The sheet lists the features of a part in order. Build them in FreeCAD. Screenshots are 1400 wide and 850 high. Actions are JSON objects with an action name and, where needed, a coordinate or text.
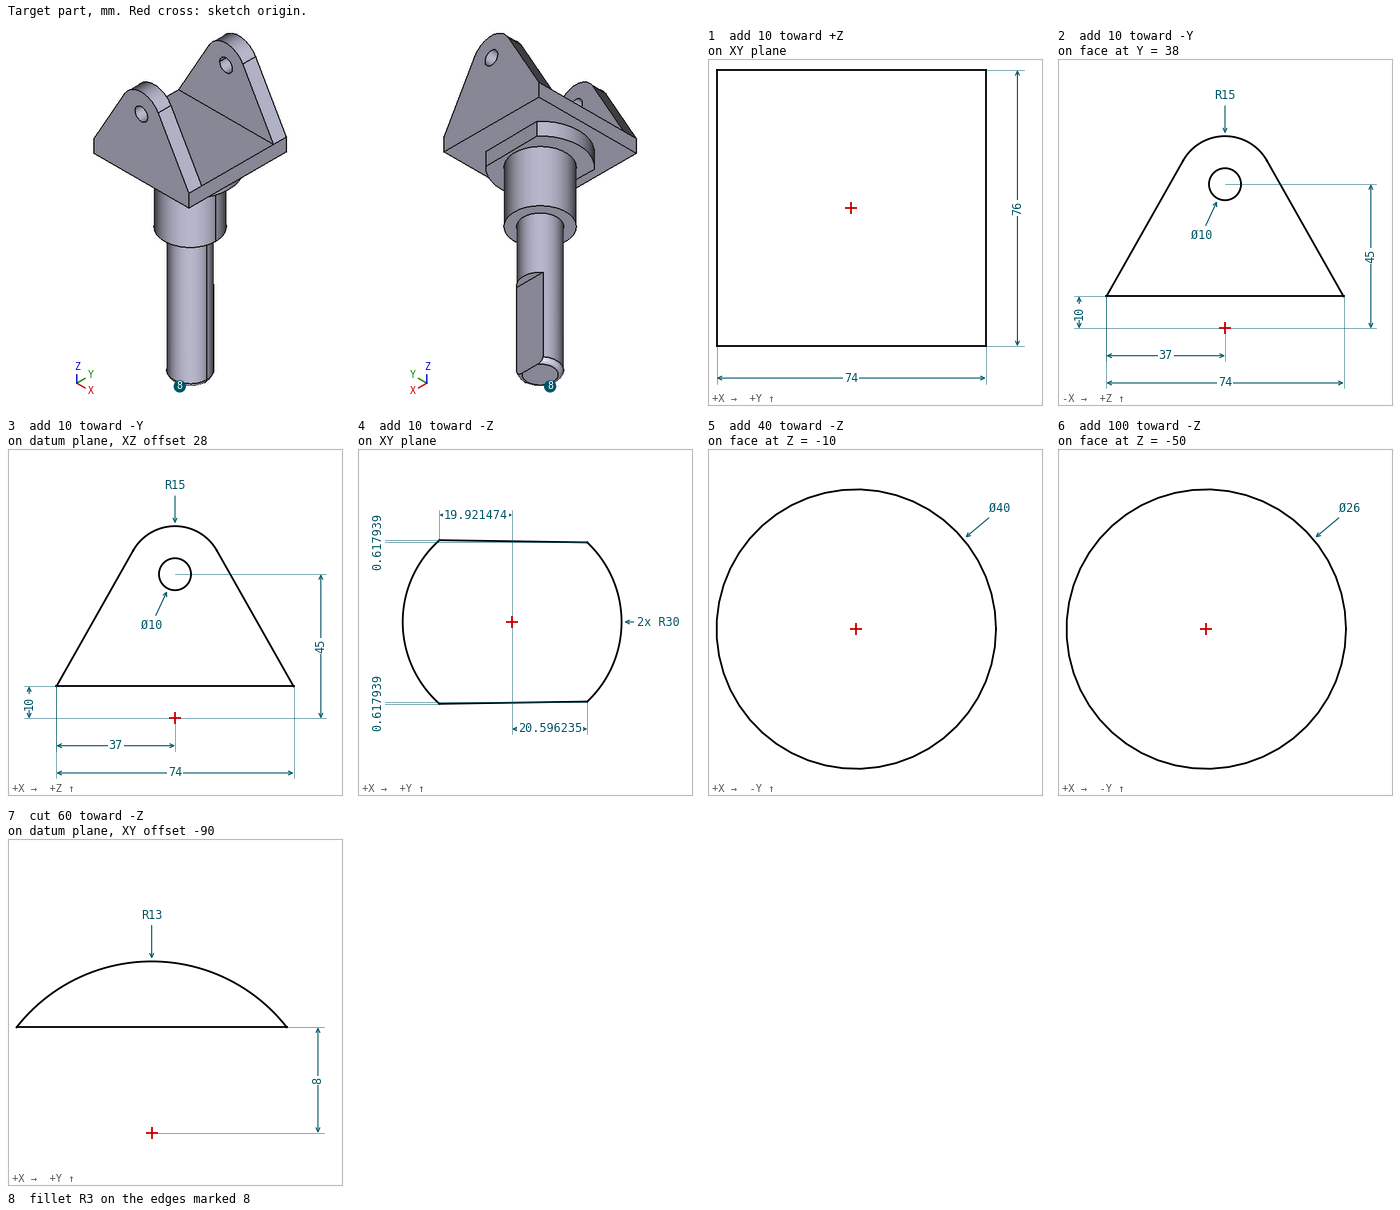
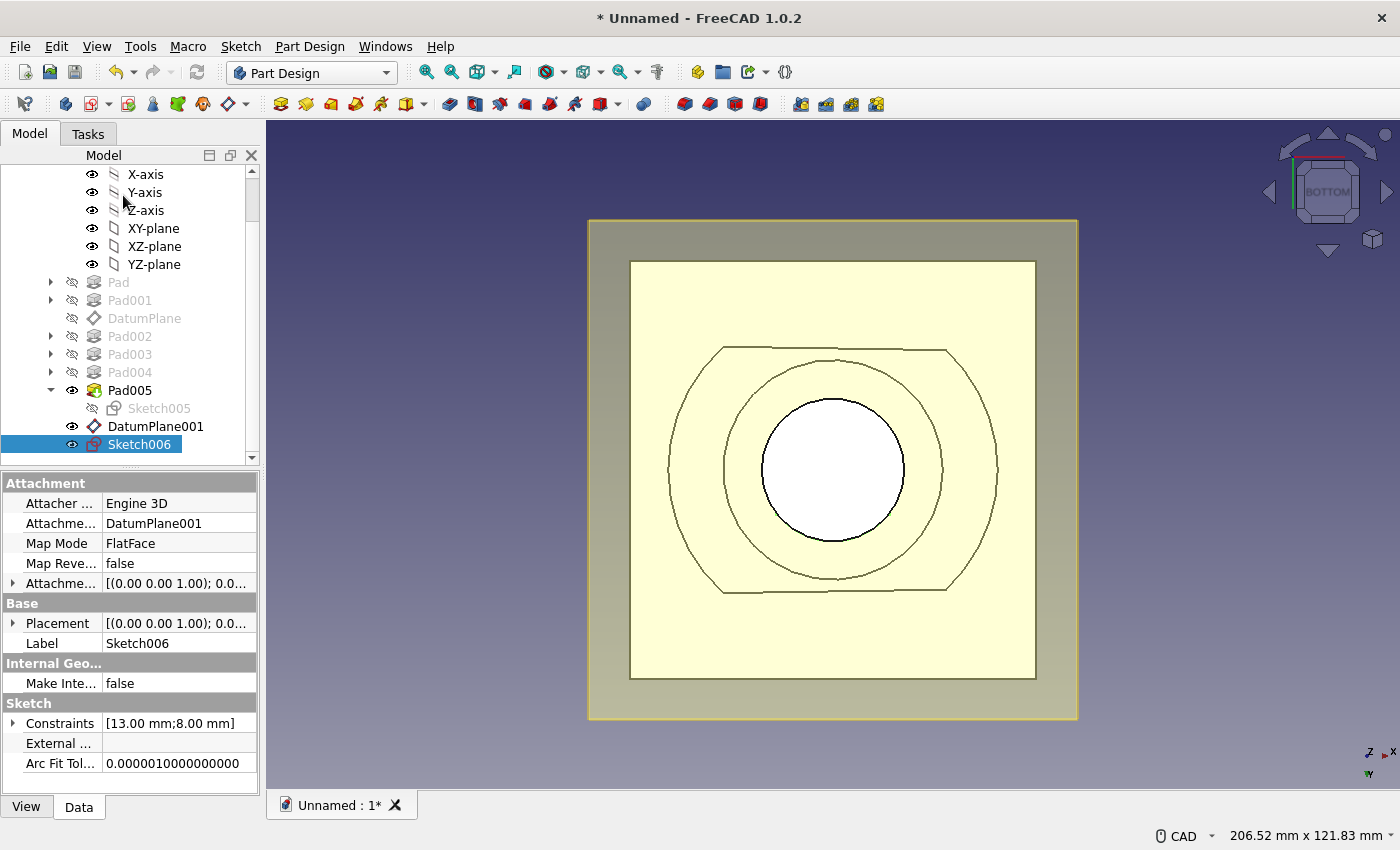
{"action": "left_click", "coordinate": [450, 104]}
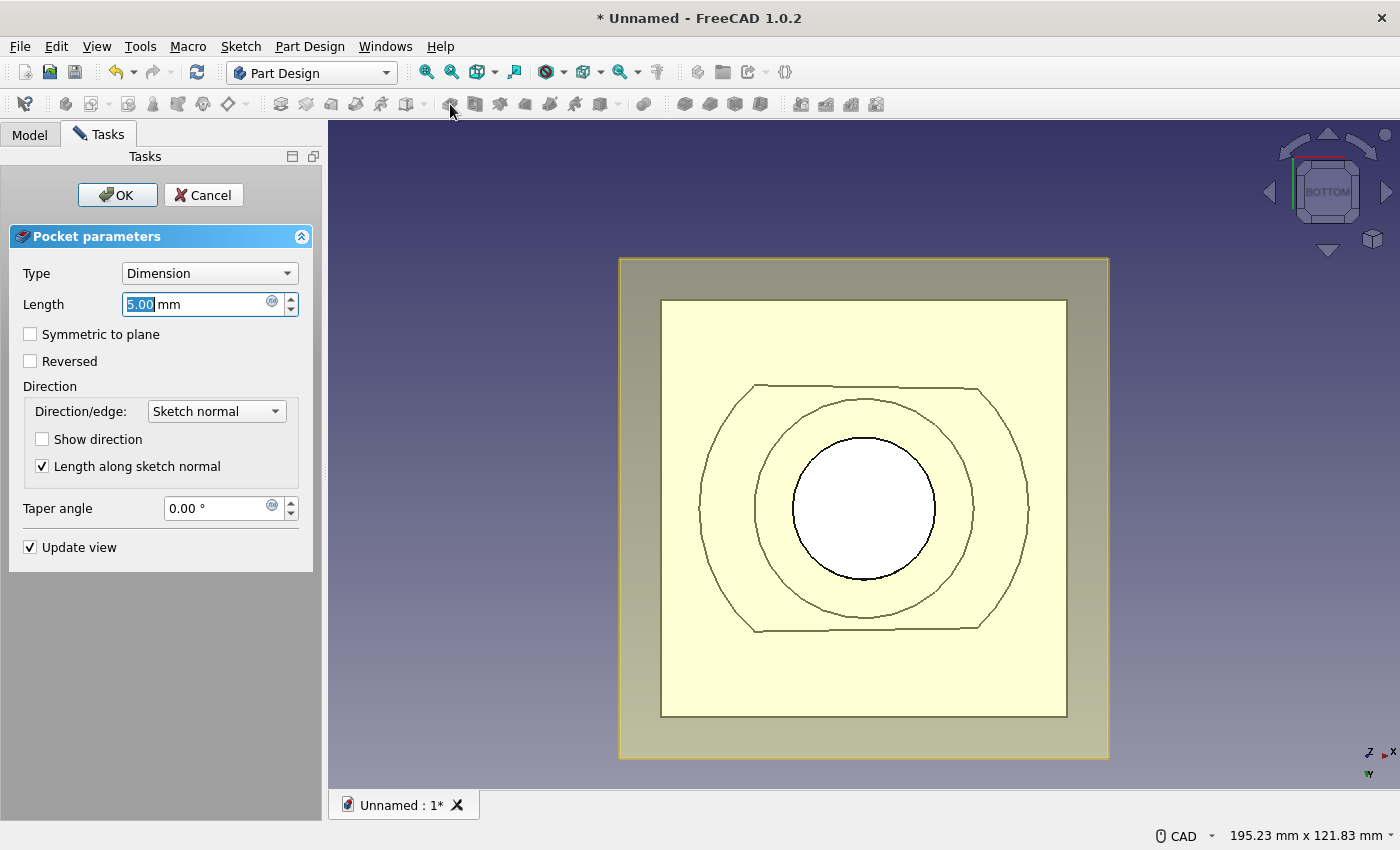
{"action": "type", "text": "60"}
{"action": "key", "text": "Tab"}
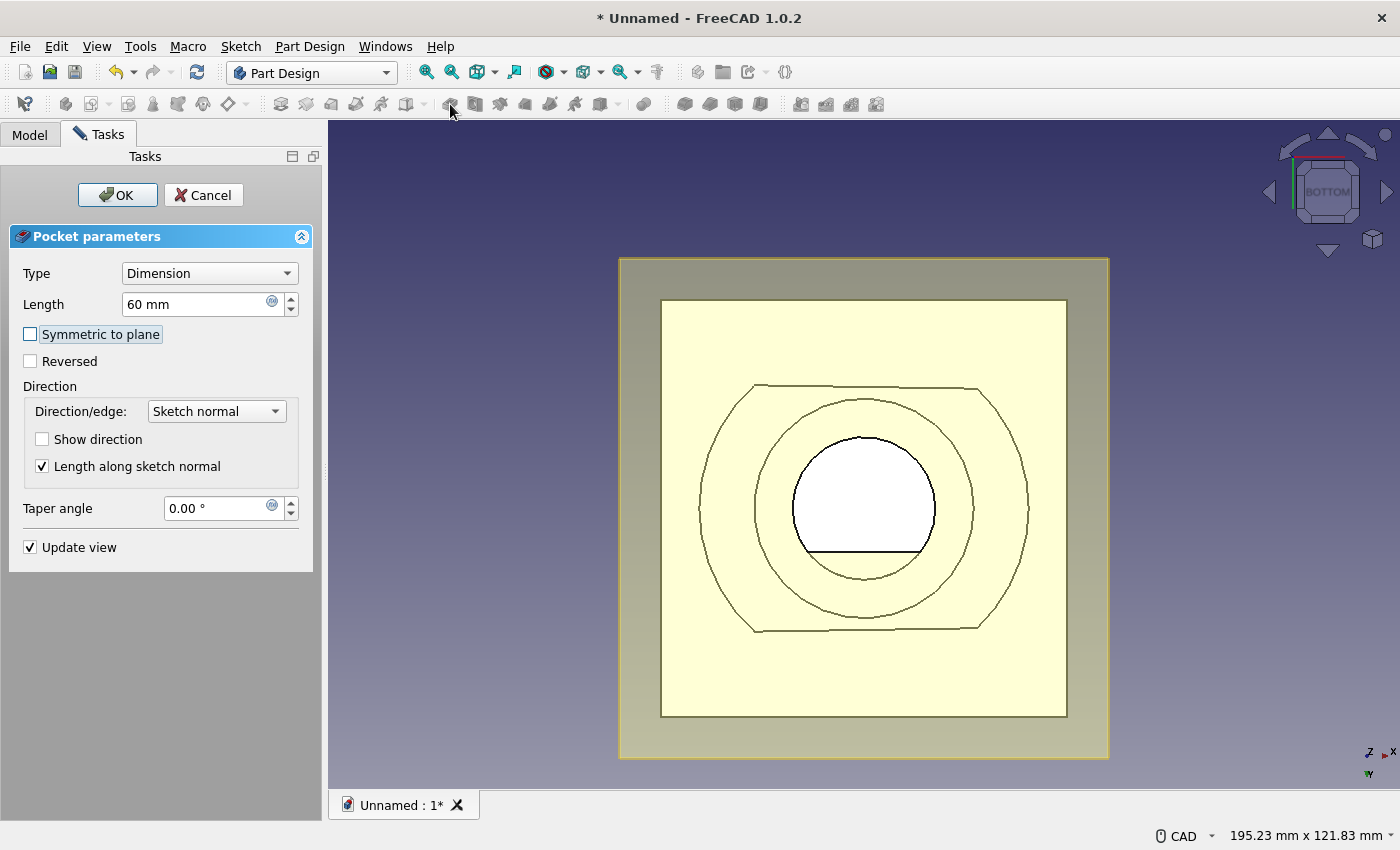
{"action": "left_click", "coordinate": [118, 195]}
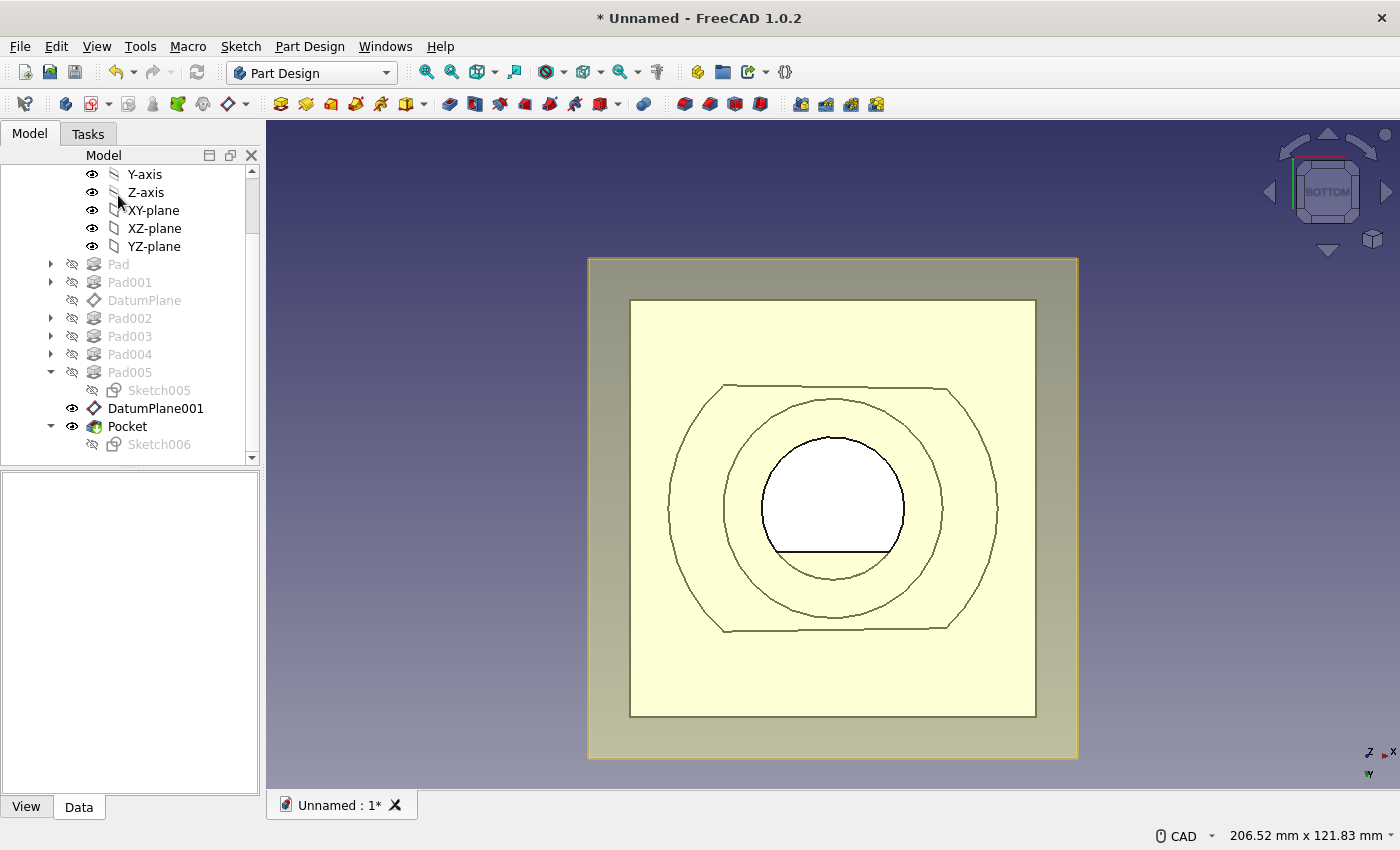
{"action": "left_click", "coordinate": [117, 408]}
{"action": "key", "text": "space"}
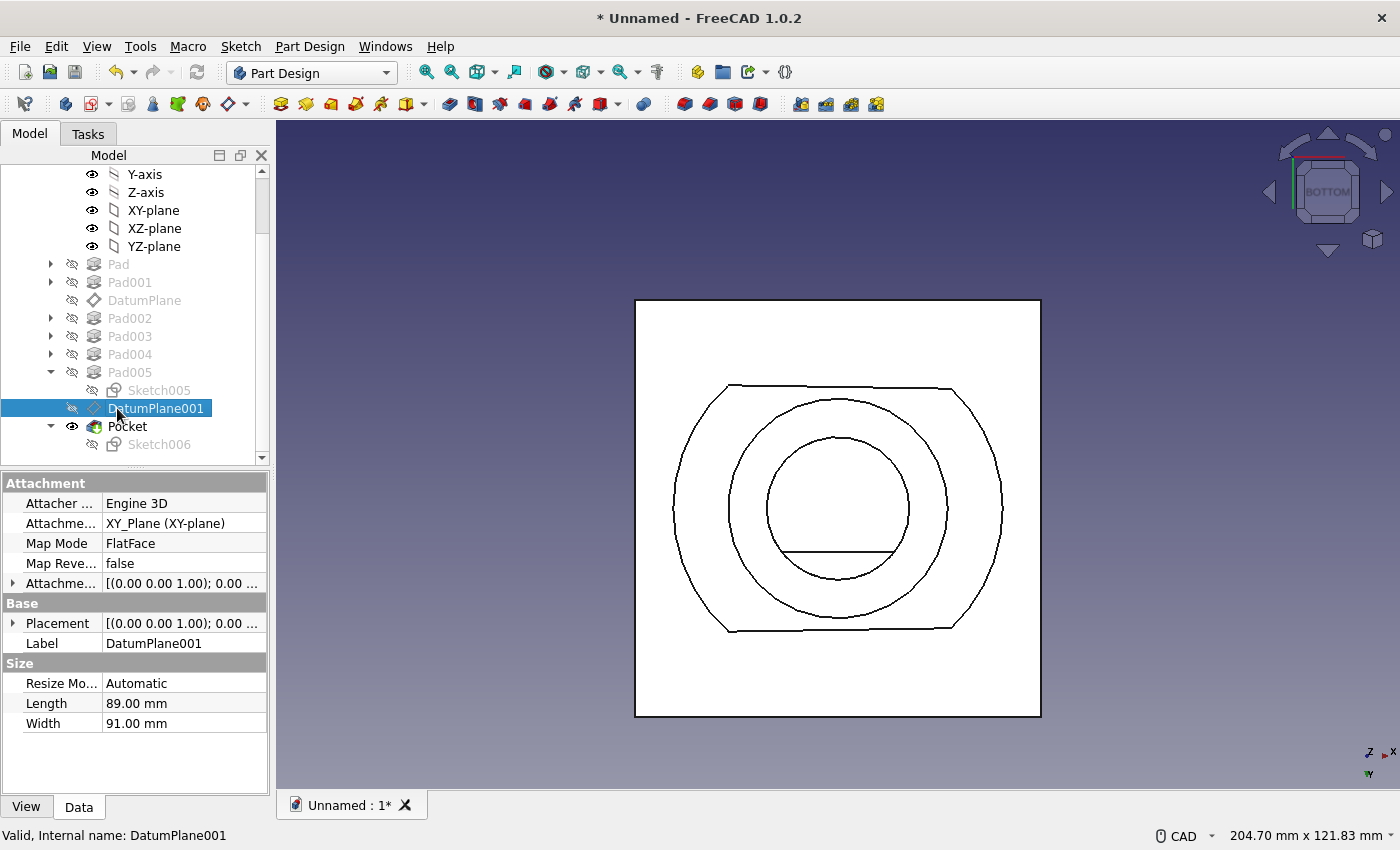
{"action": "left_click", "coordinate": [890, 458]}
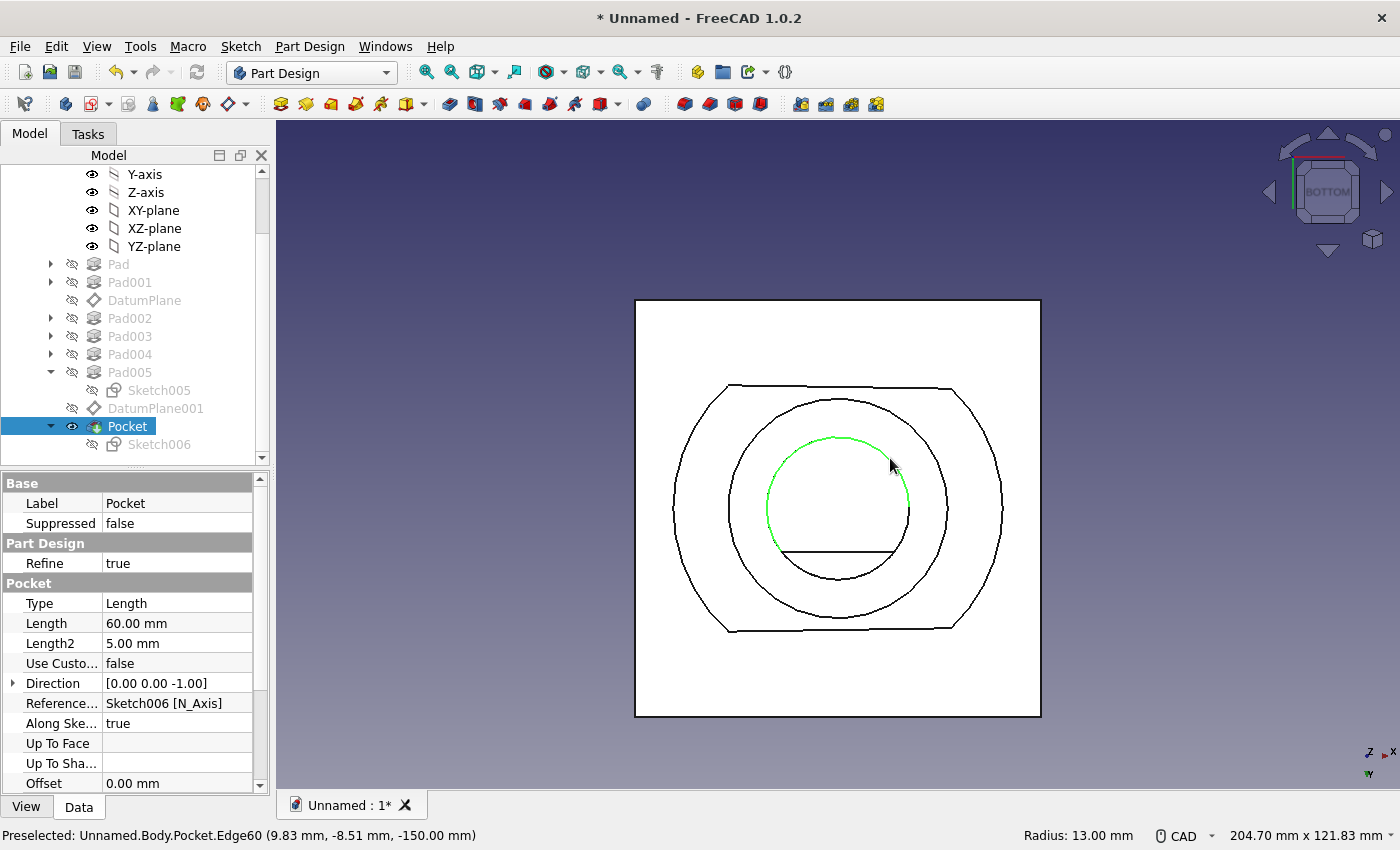
{"action": "left_click", "coordinate": [685, 104]}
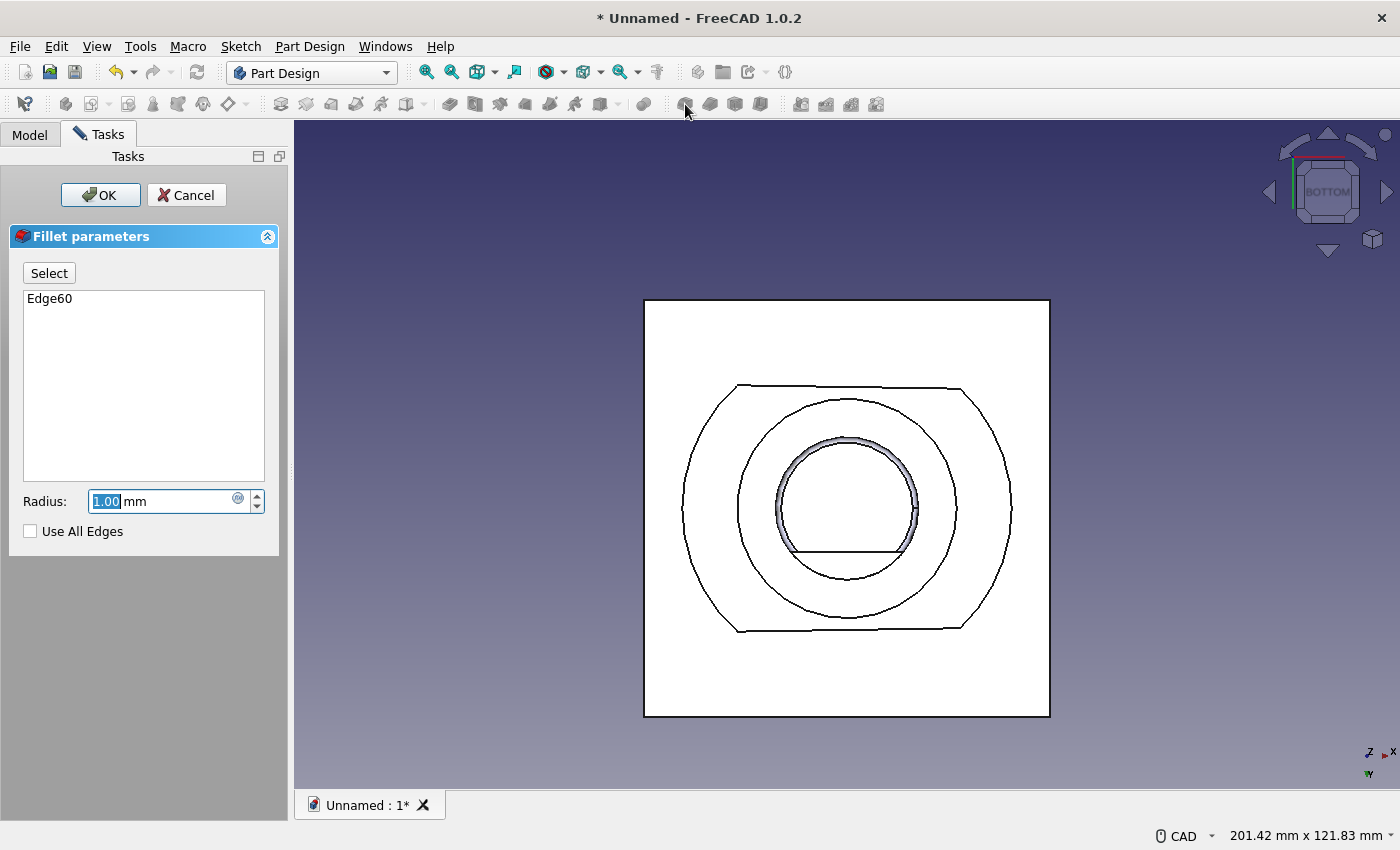
{"action": "type", "text": "3"}
{"action": "key", "text": "Tab"}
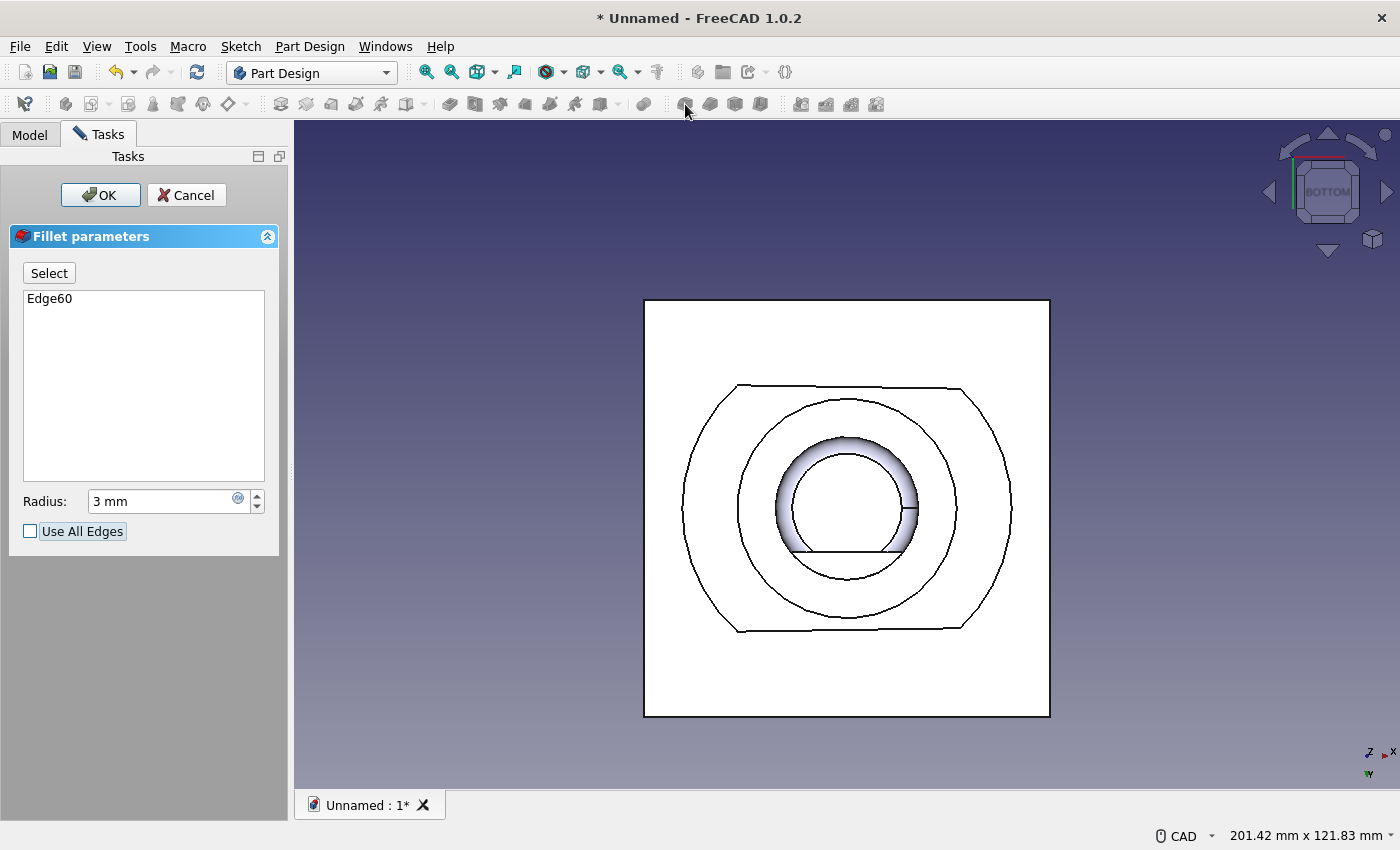
{"action": "left_click", "coordinate": [101, 195]}